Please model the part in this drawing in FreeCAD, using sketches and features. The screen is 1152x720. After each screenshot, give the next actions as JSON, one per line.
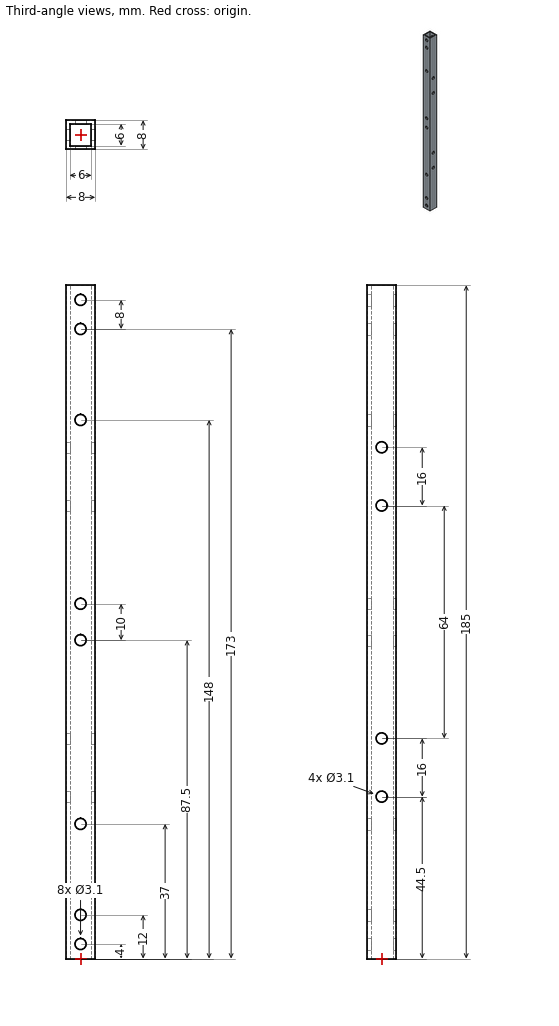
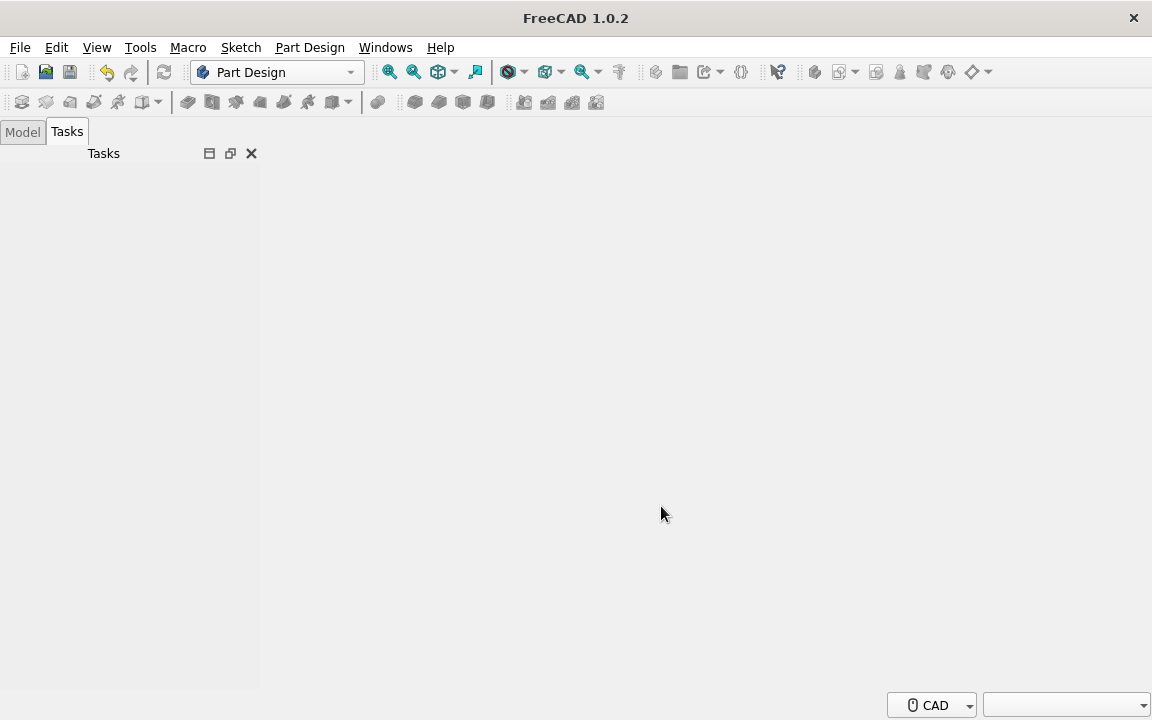
{"action": "left_click", "coordinate": [22, 72]}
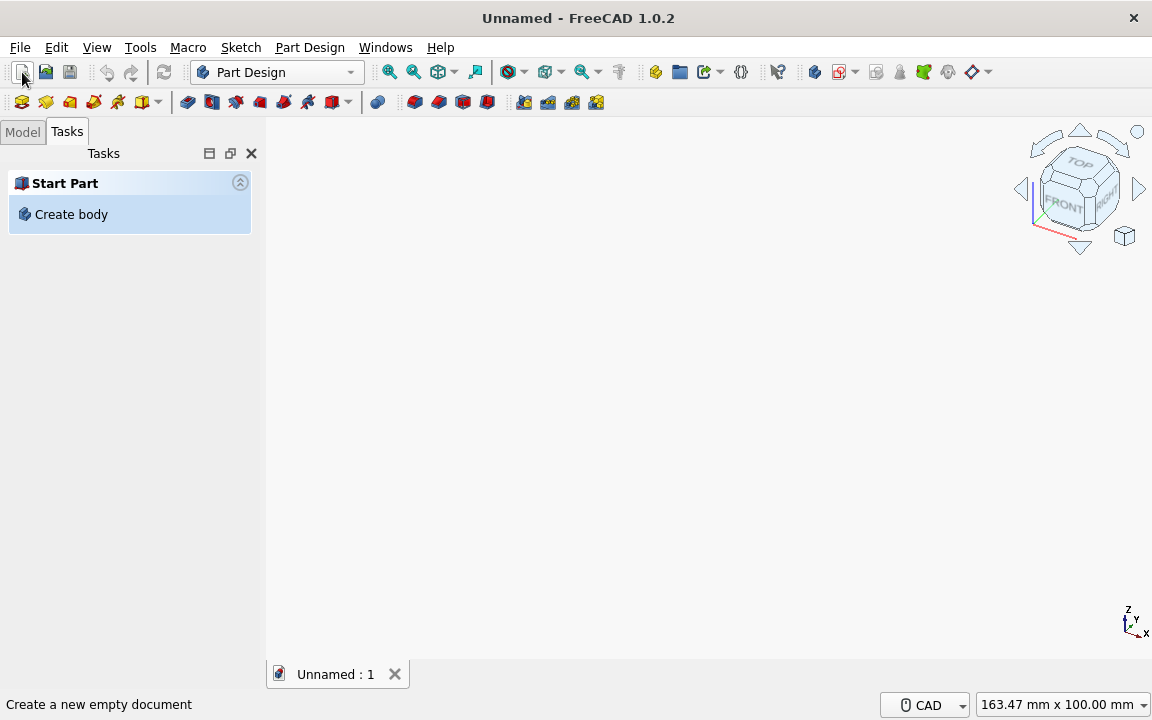
{"action": "left_click", "coordinate": [840, 72]}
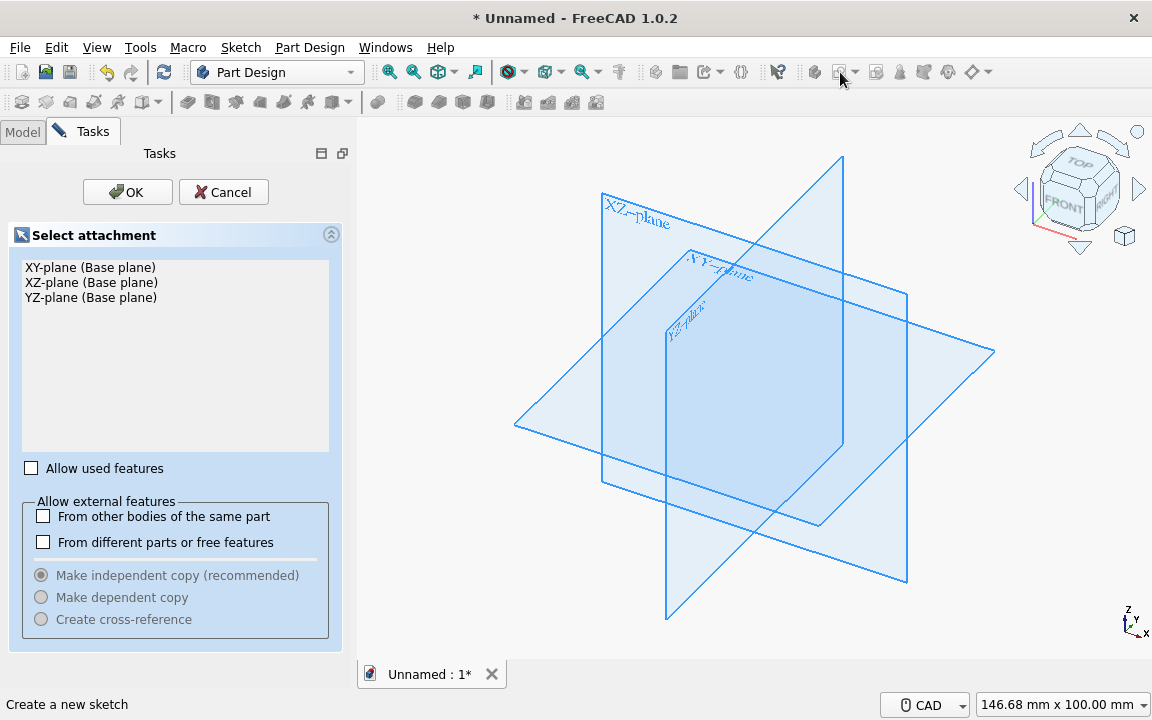
{"action": "left_click", "coordinate": [82, 268]}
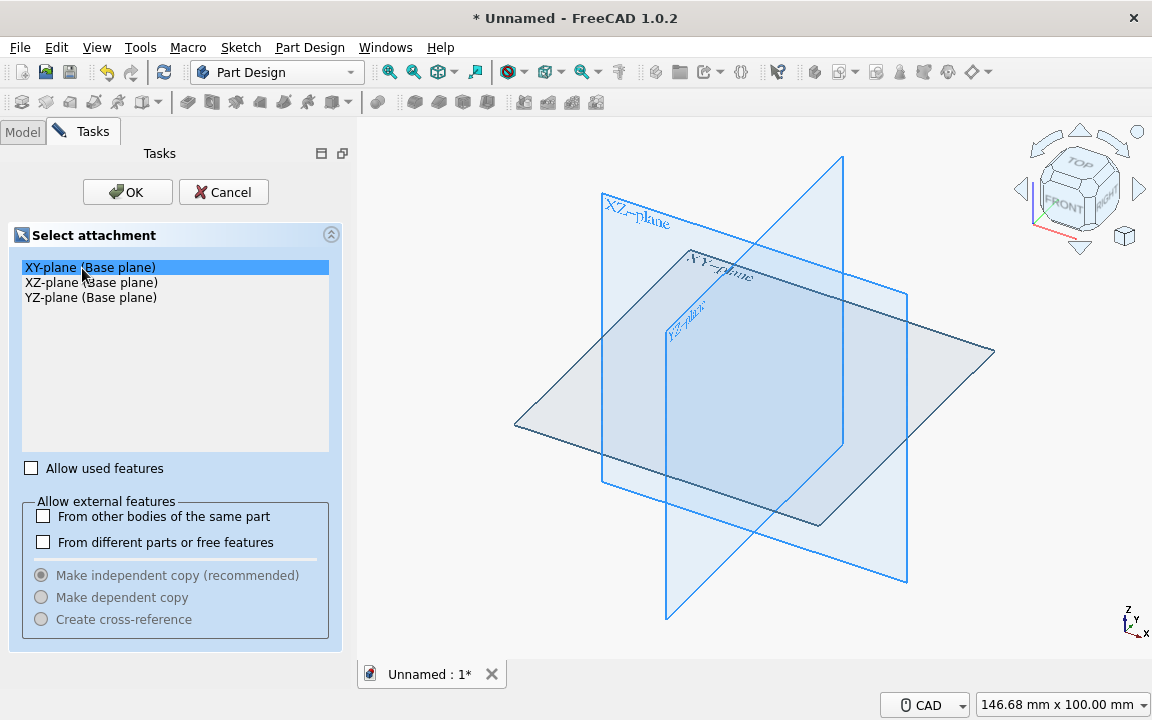
{"action": "left_click", "coordinate": [128, 192]}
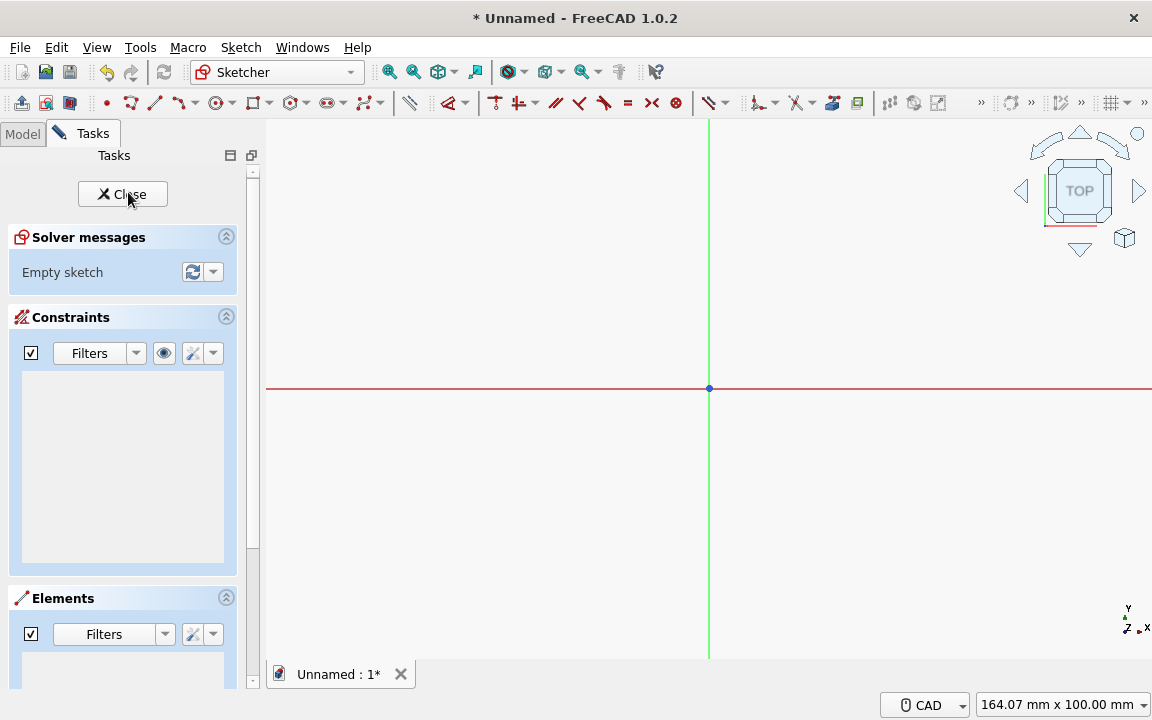
{"action": "scroll", "coordinate": [720, 389], "scroll_direction": "up", "scroll_amount": 10}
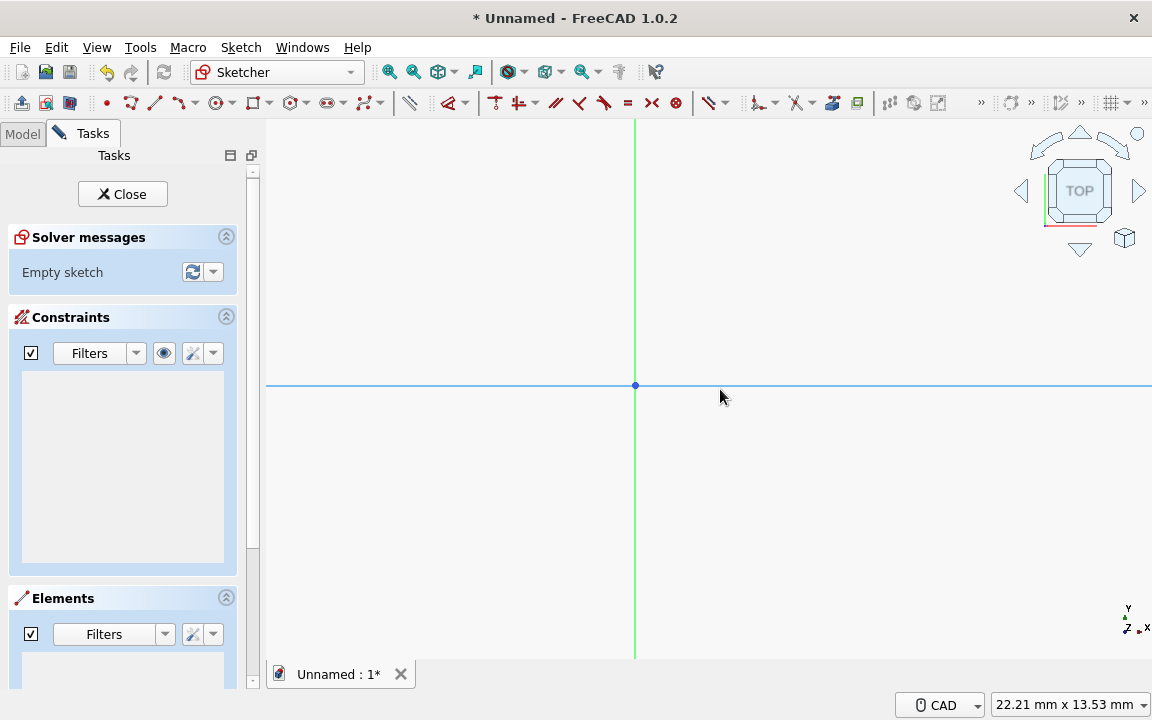
{"action": "key", "text": "g v"}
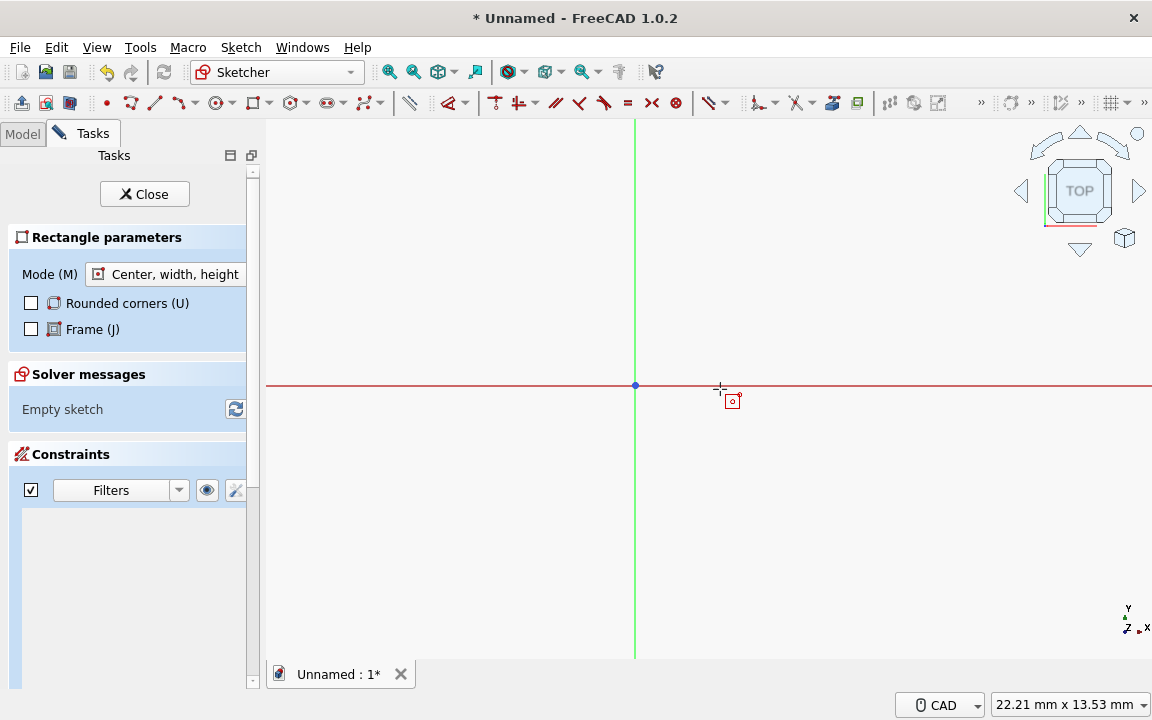
{"action": "left_click", "coordinate": [635, 386]}
{"action": "left_click", "coordinate": [795, 226]}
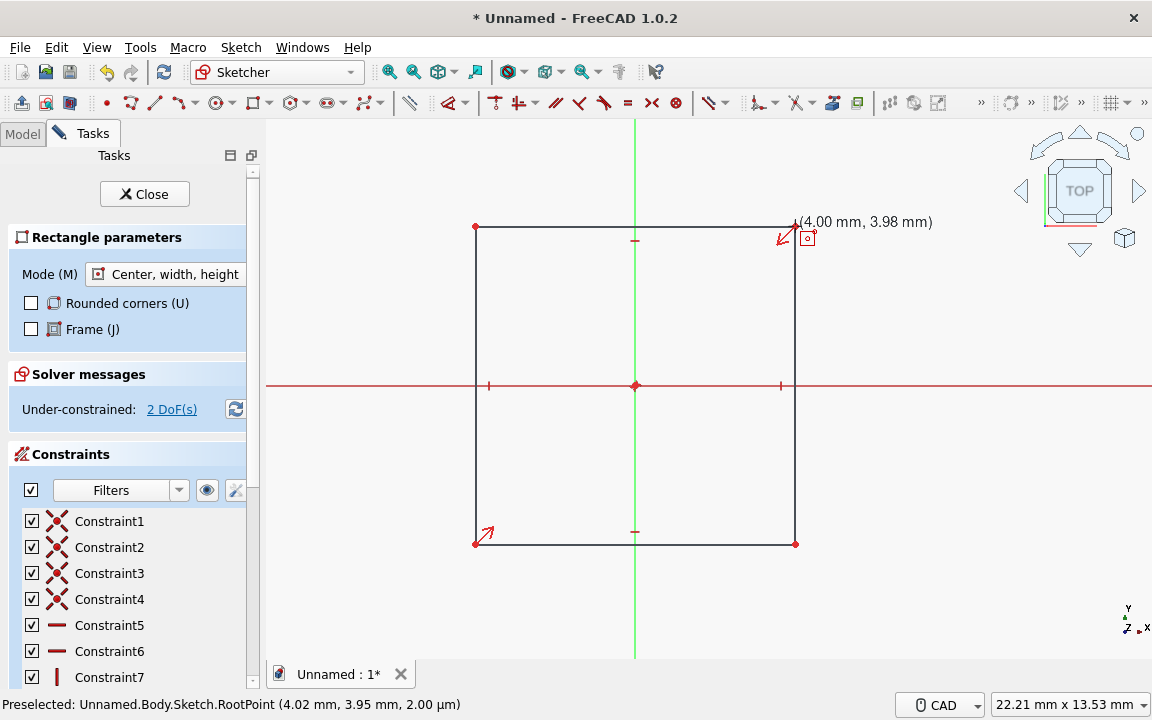
{"action": "left_click", "coordinate": [635, 386]}
{"action": "left_click", "coordinate": [755, 266]}
{"action": "key", "text": "Escape"}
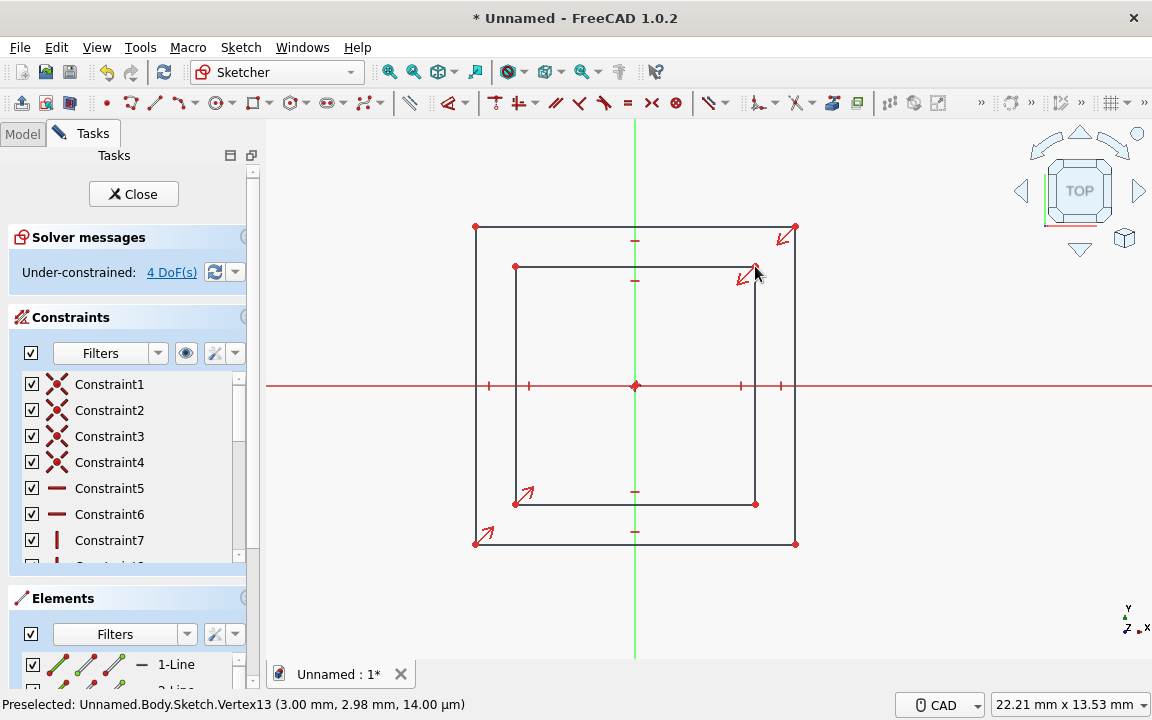
{"action": "left_click", "coordinate": [448, 104]}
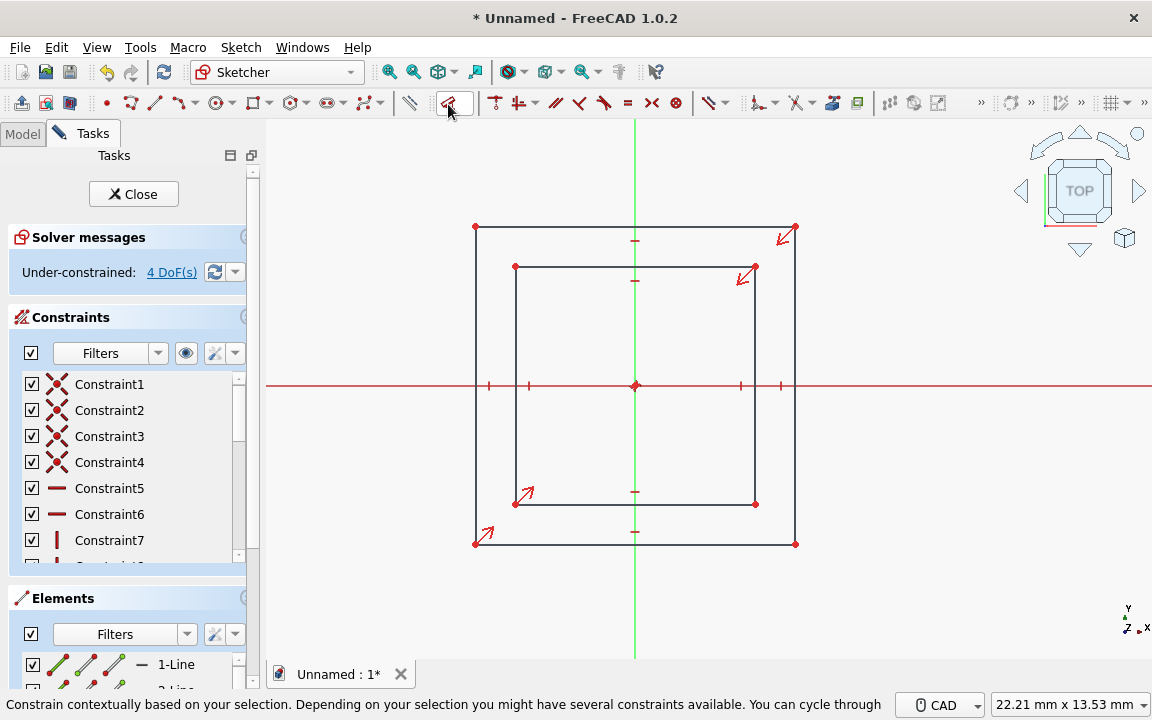
{"action": "left_click", "coordinate": [572, 545]}
{"action": "left_click", "coordinate": [562, 579]}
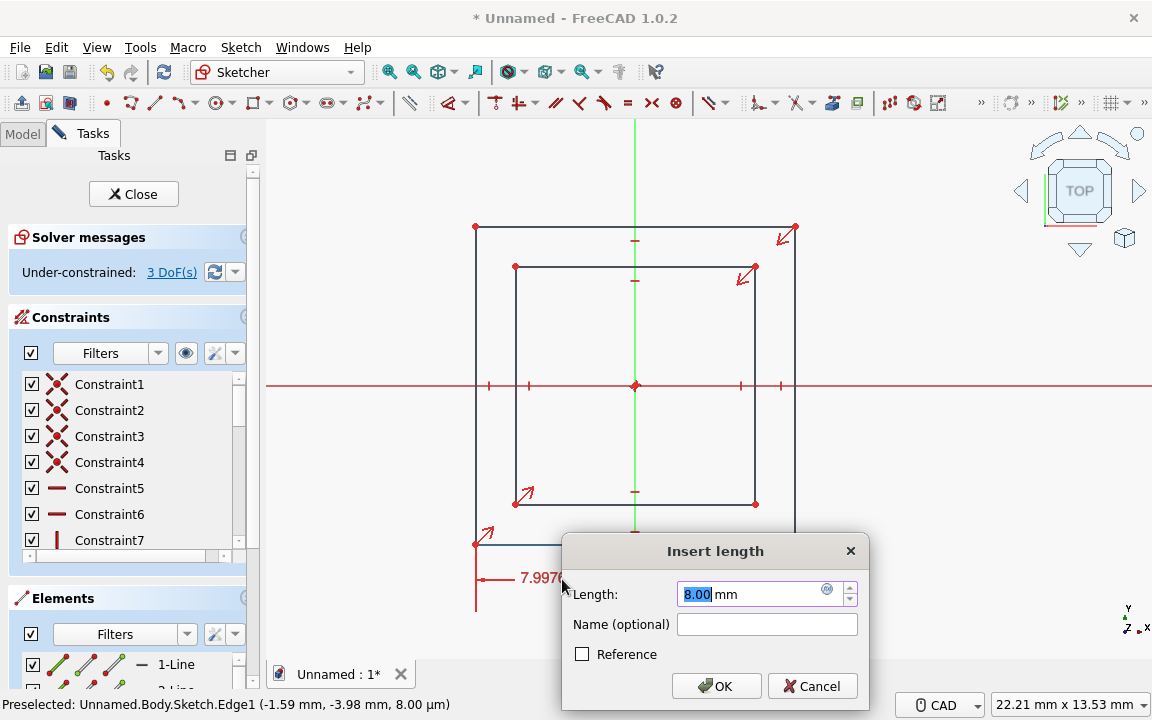
{"action": "type", "text": "8"}
{"action": "key", "text": "Return"}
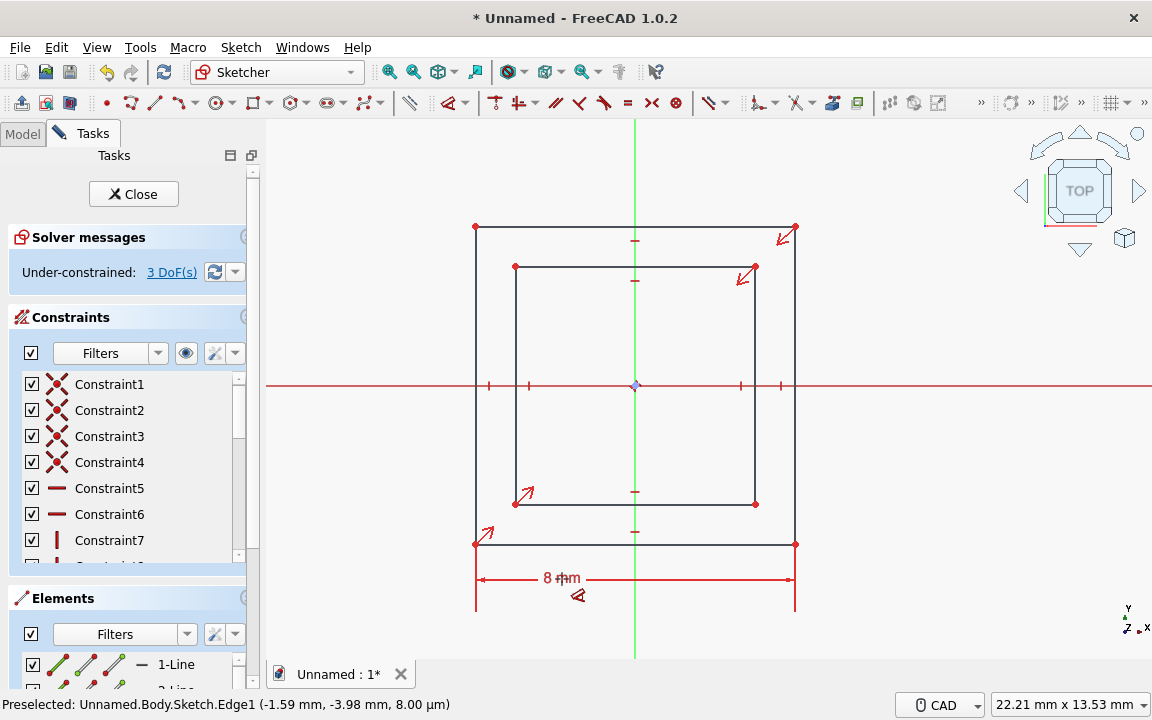
{"action": "left_click", "coordinate": [795, 449]}
{"action": "left_click", "coordinate": [829, 313]}